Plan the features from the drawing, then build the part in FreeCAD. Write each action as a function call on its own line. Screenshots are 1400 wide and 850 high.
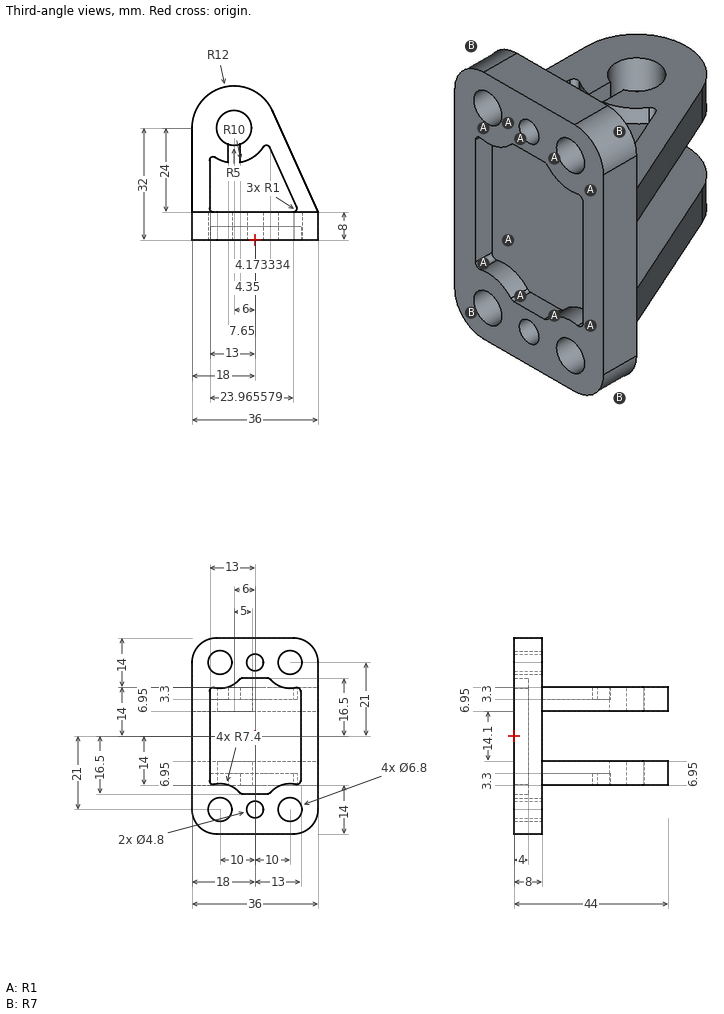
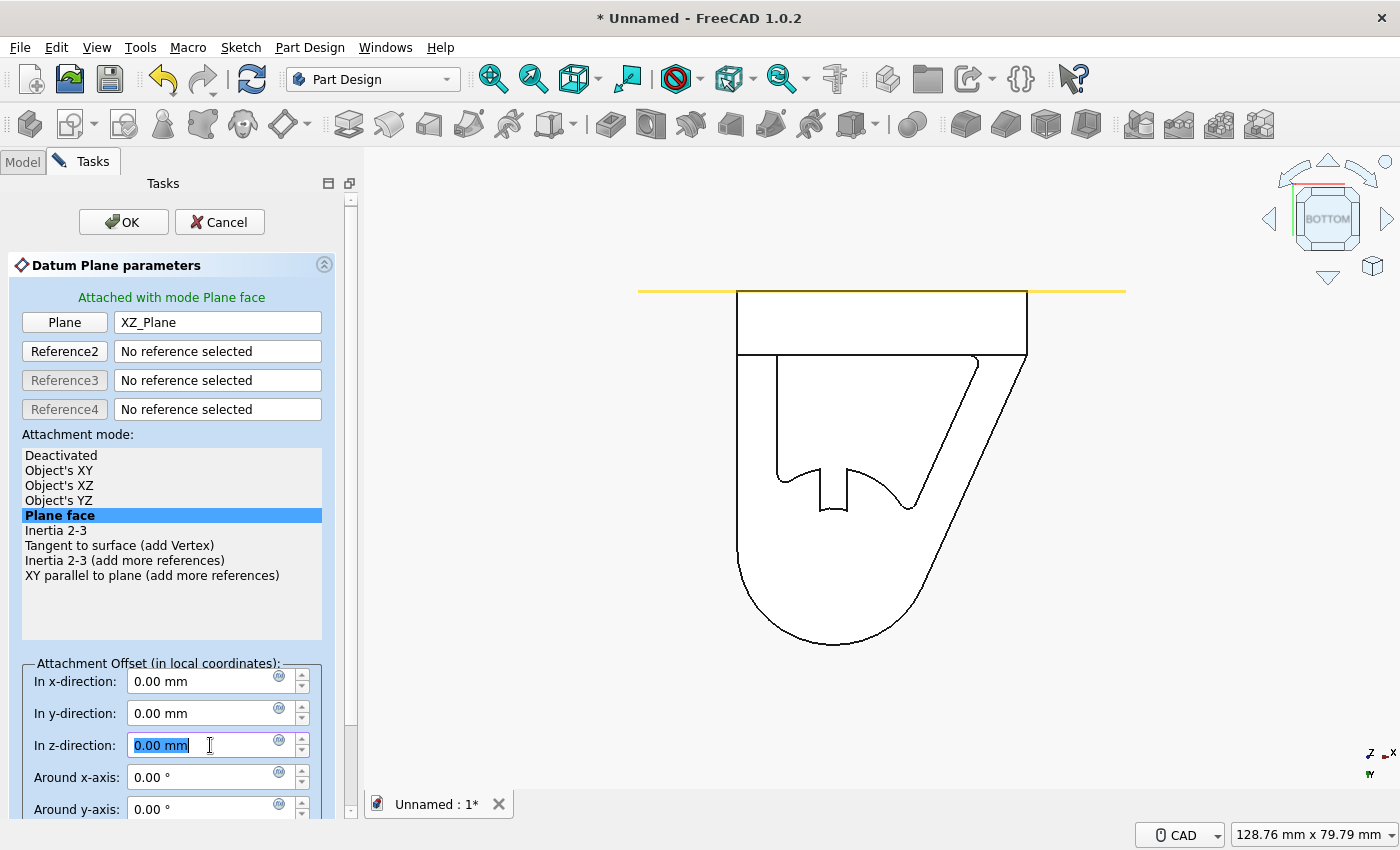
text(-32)
key(Tab)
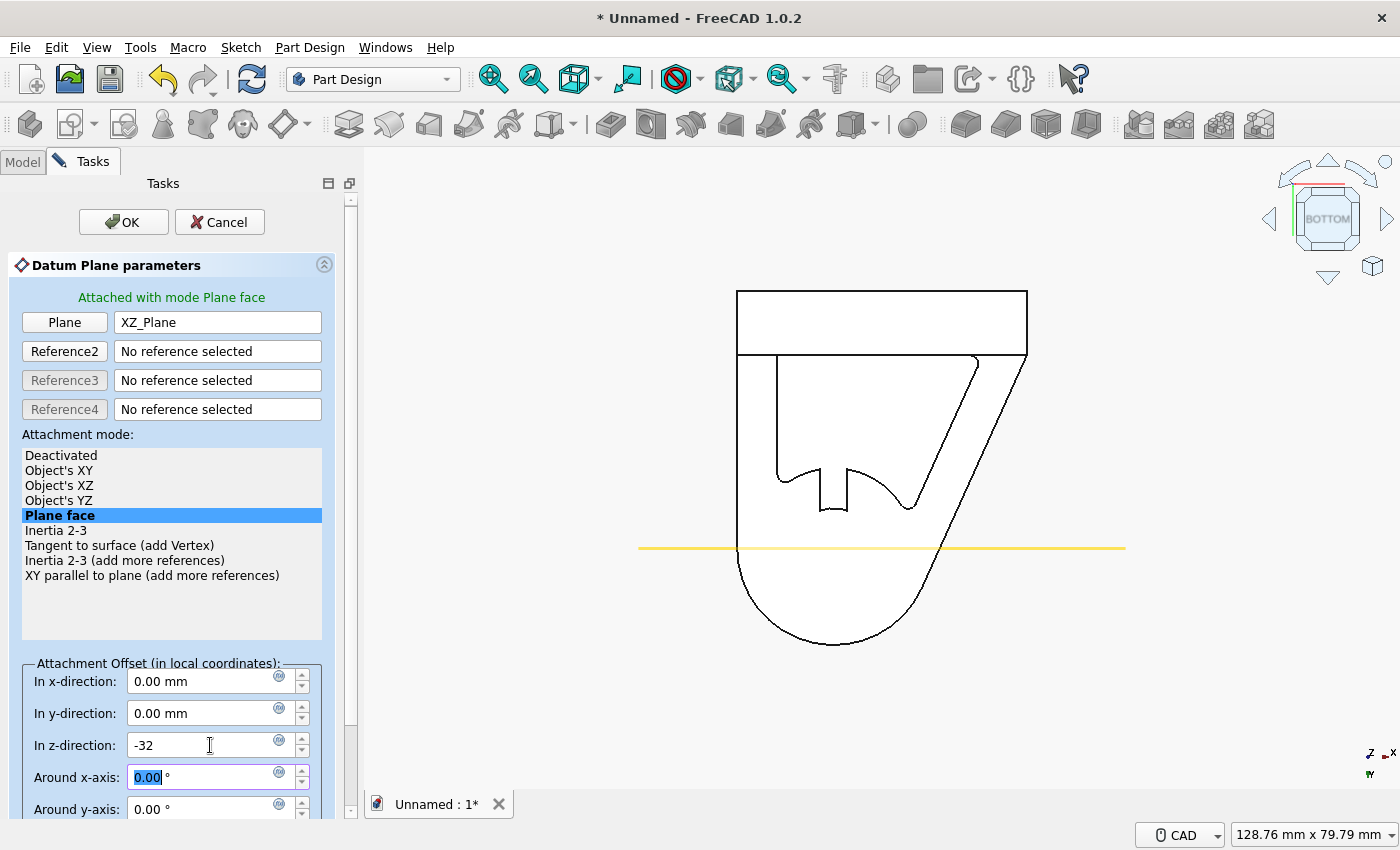
click(124, 222)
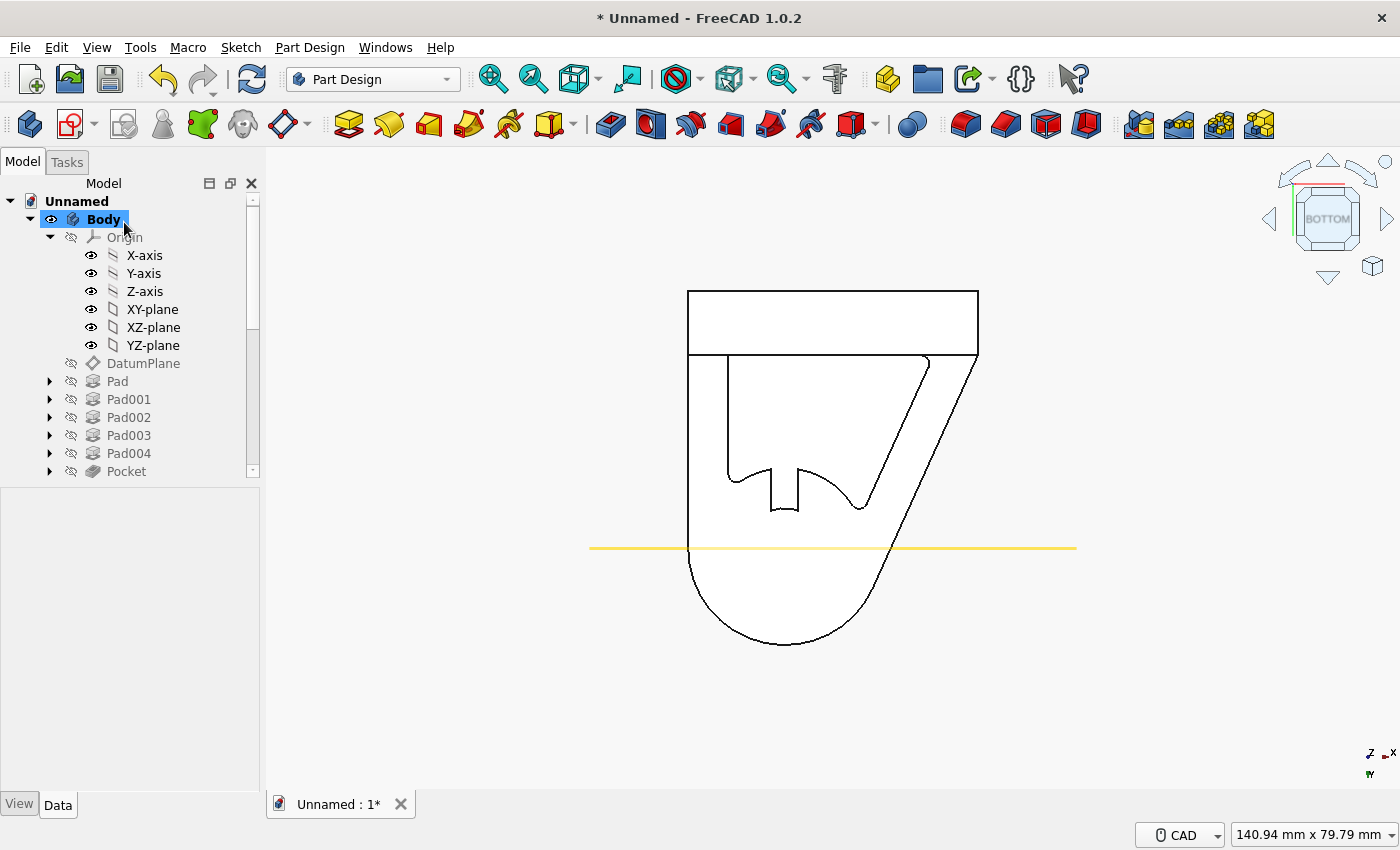
scroll(100, 341, down, 3)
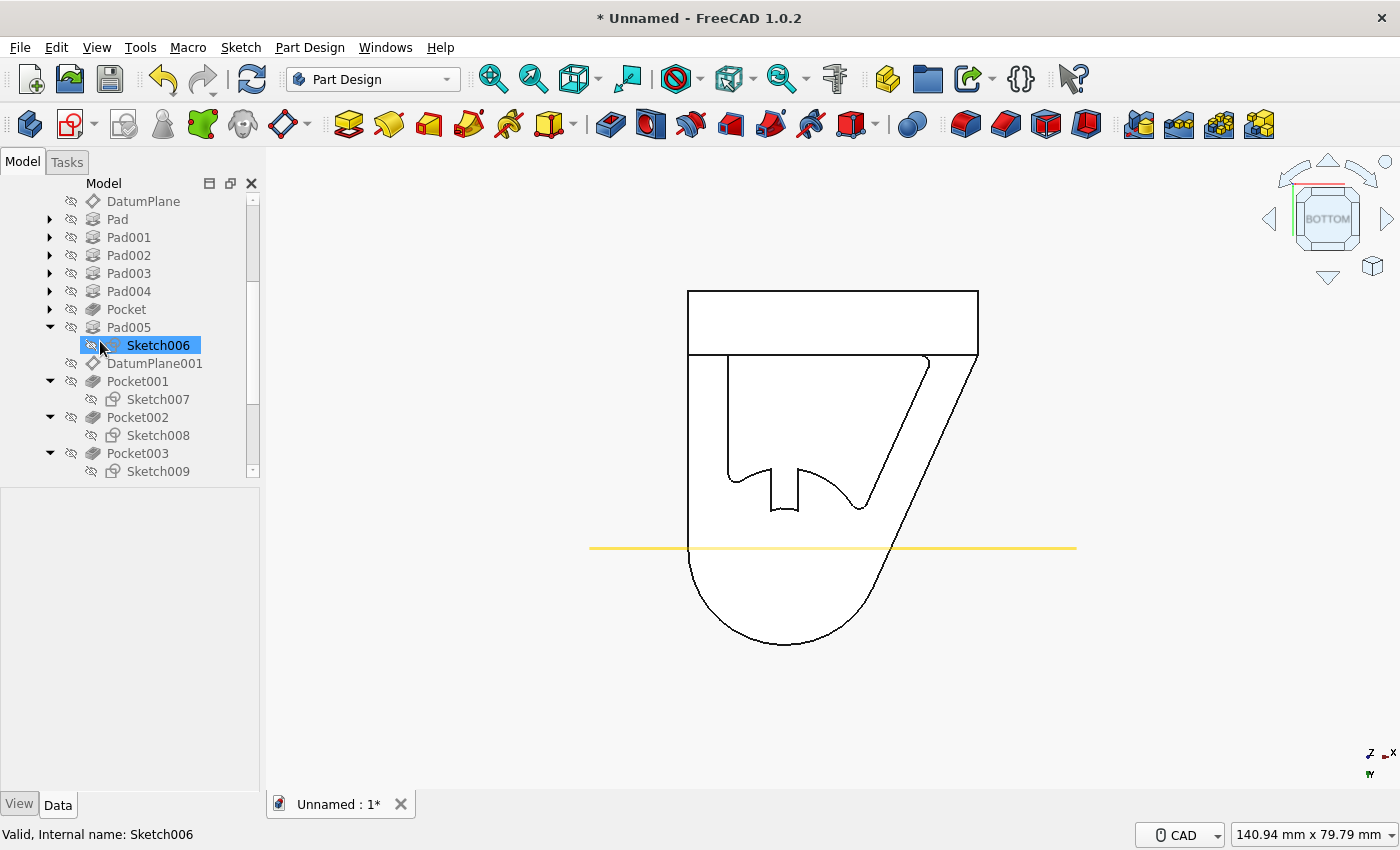
scroll(140, 341, up, 15)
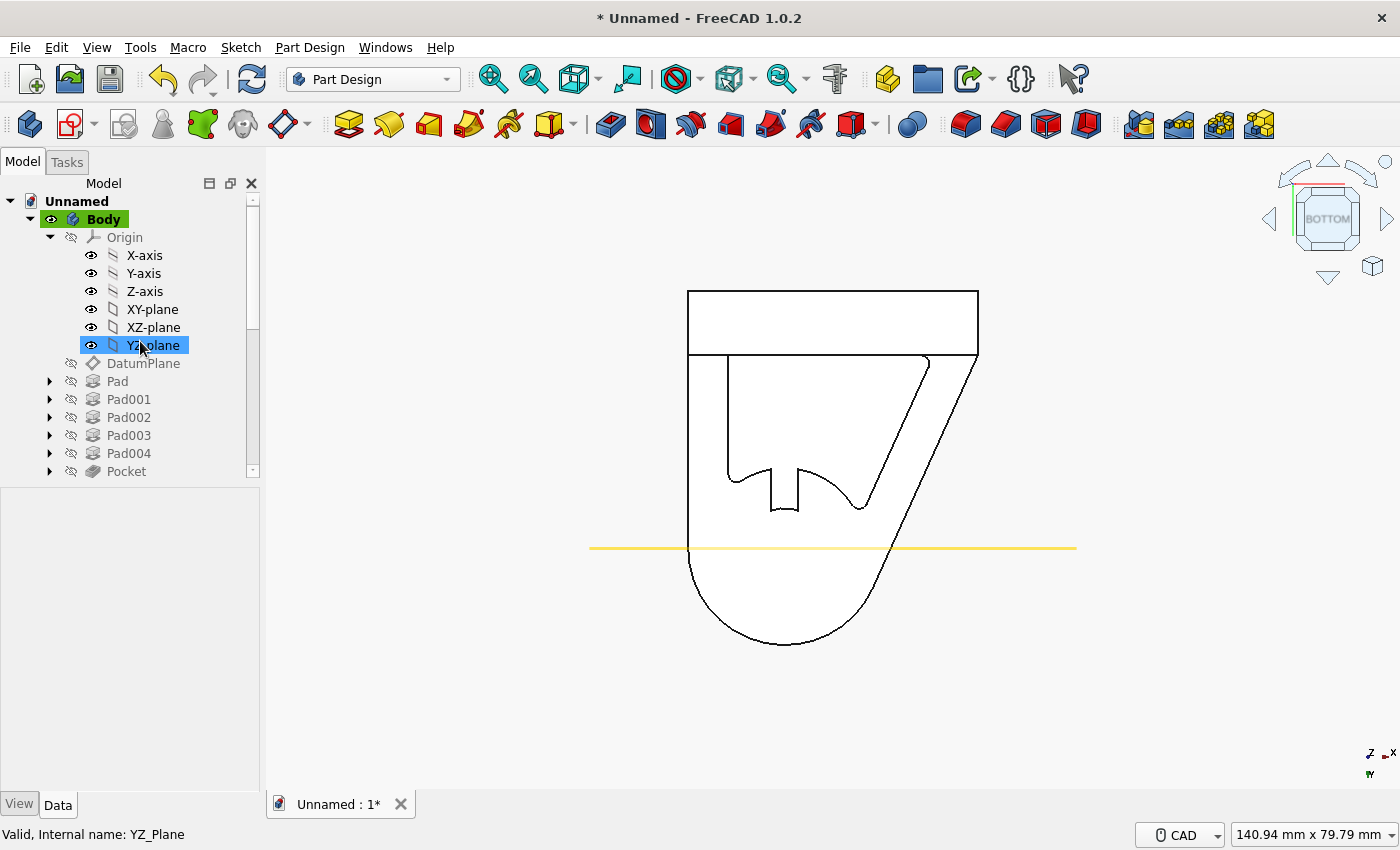
scroll(100, 341, down, 6)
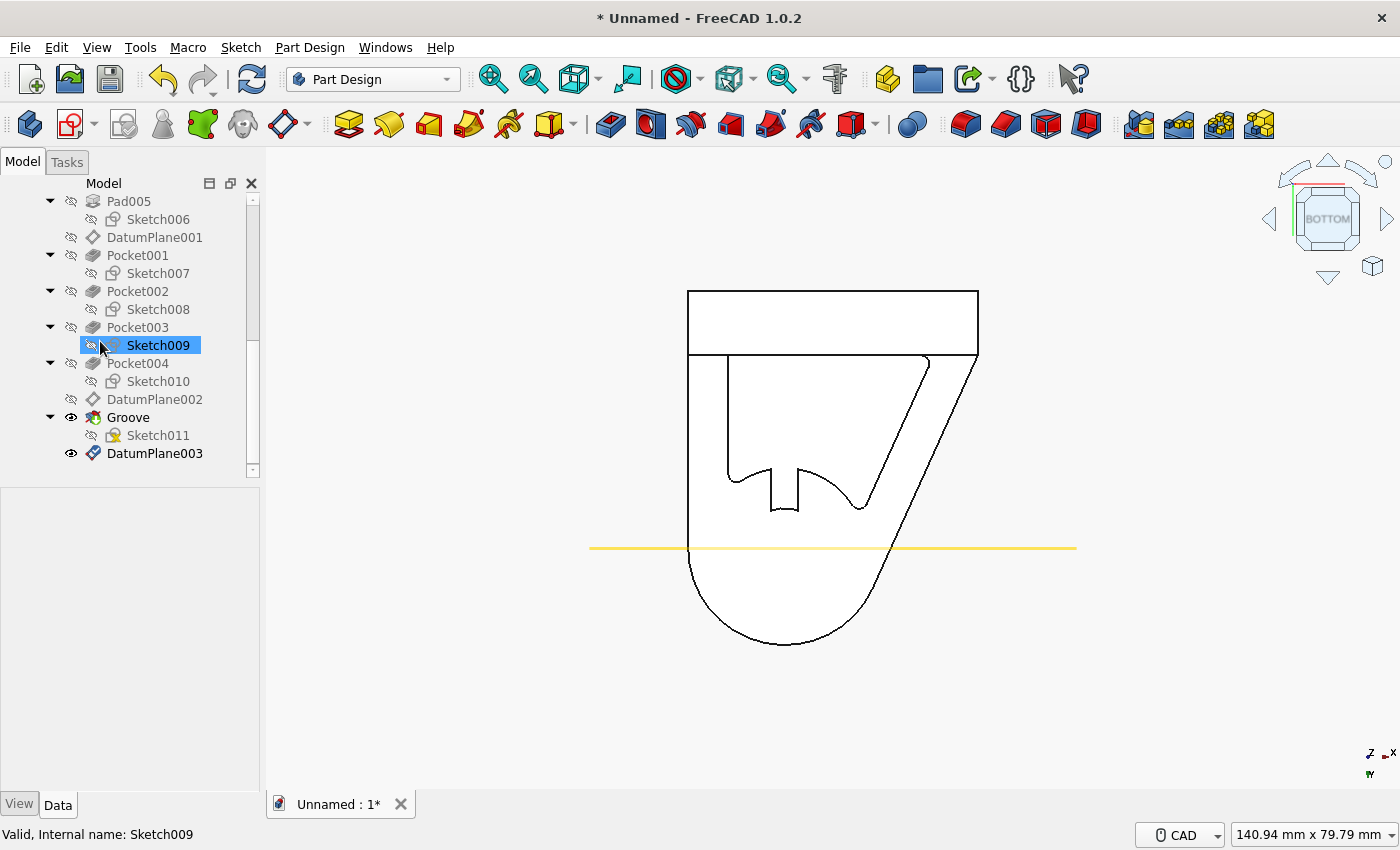
click(116, 453)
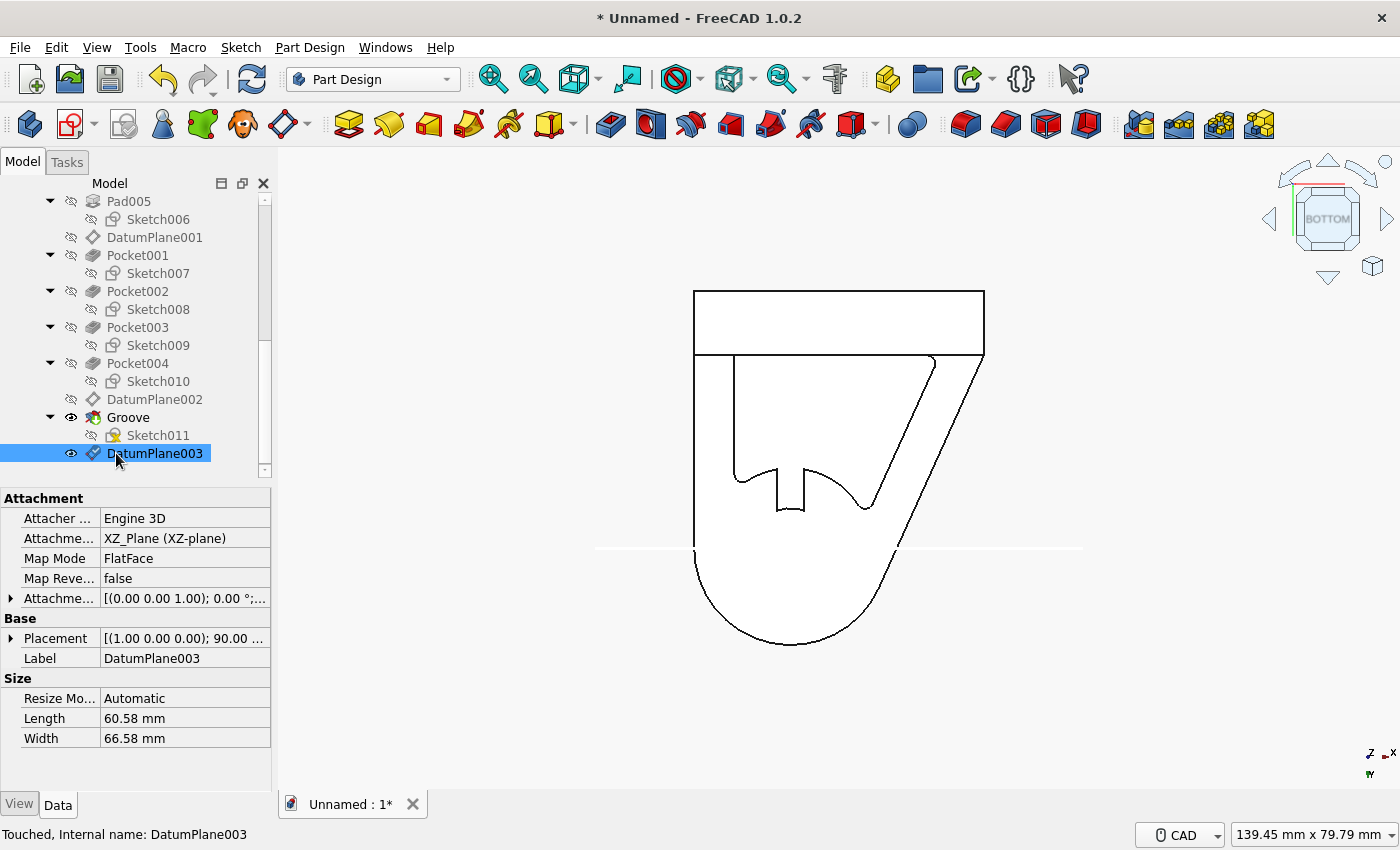
click(70, 124)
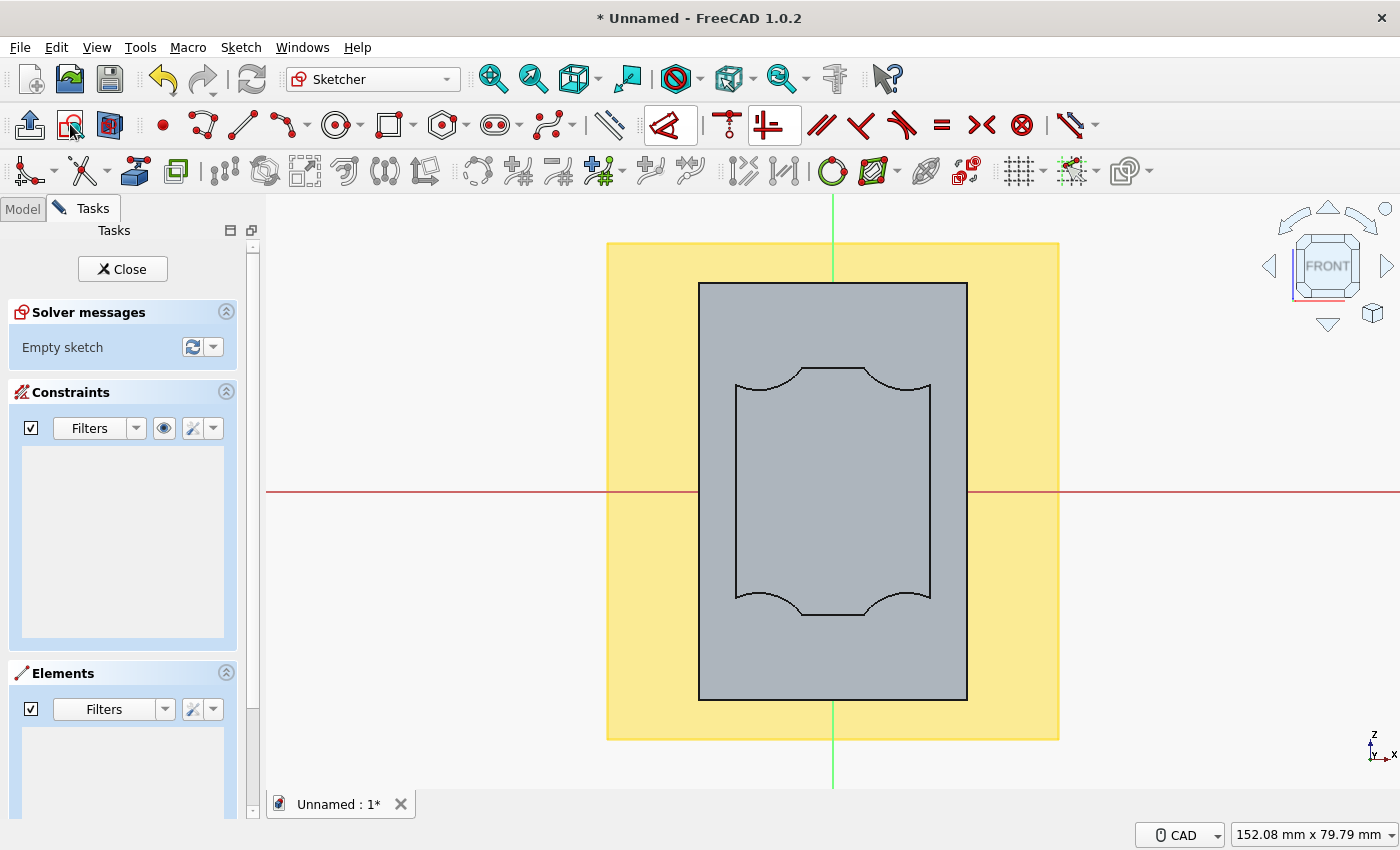
key(q)
key(s)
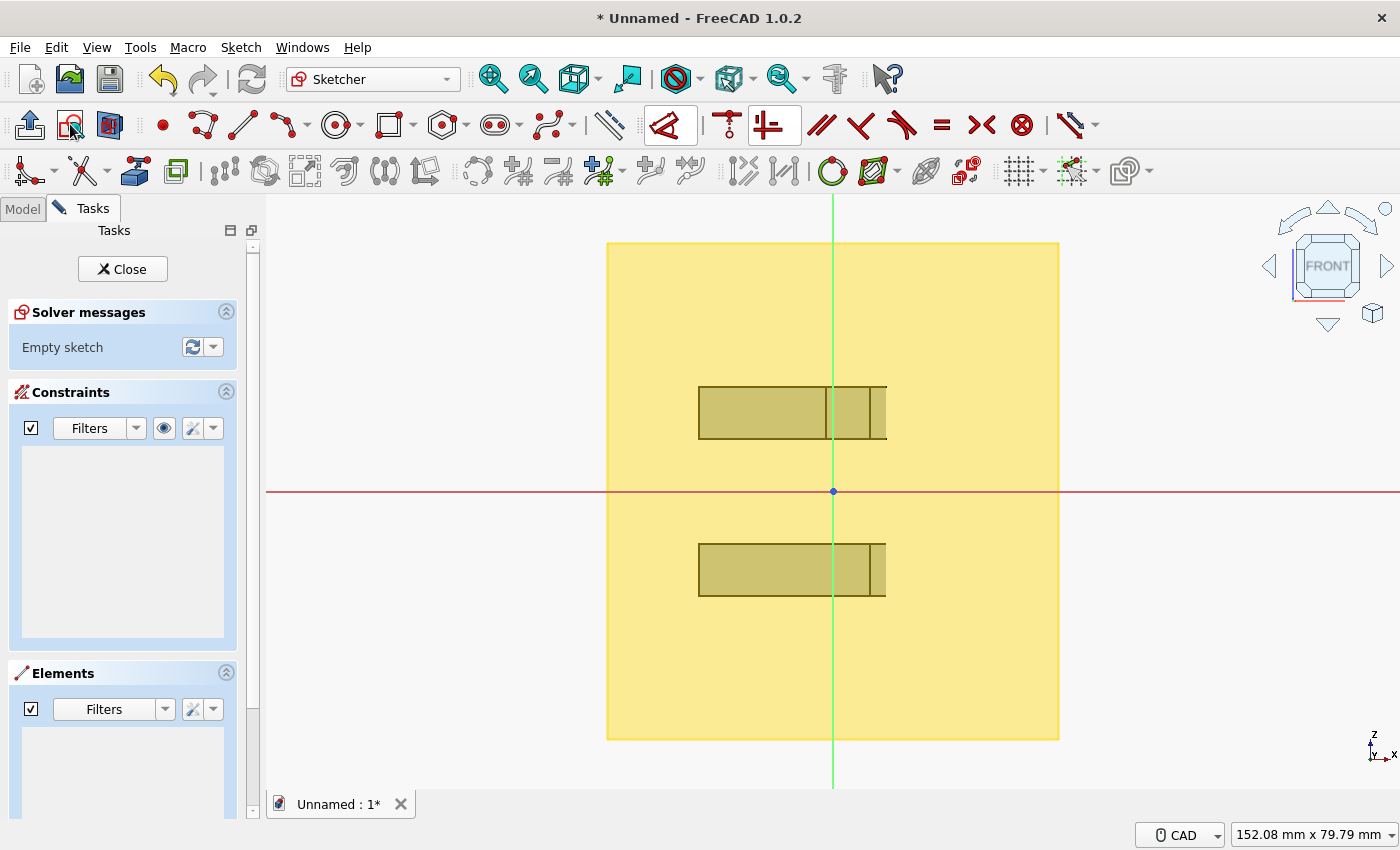
scroll(831, 581, up, 6)